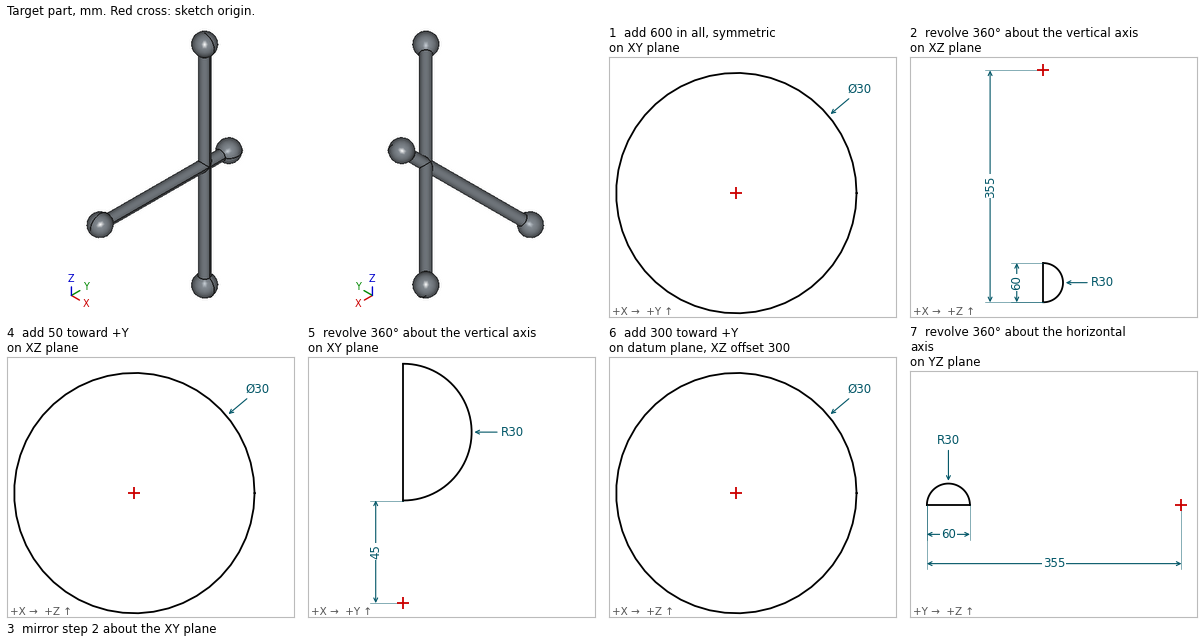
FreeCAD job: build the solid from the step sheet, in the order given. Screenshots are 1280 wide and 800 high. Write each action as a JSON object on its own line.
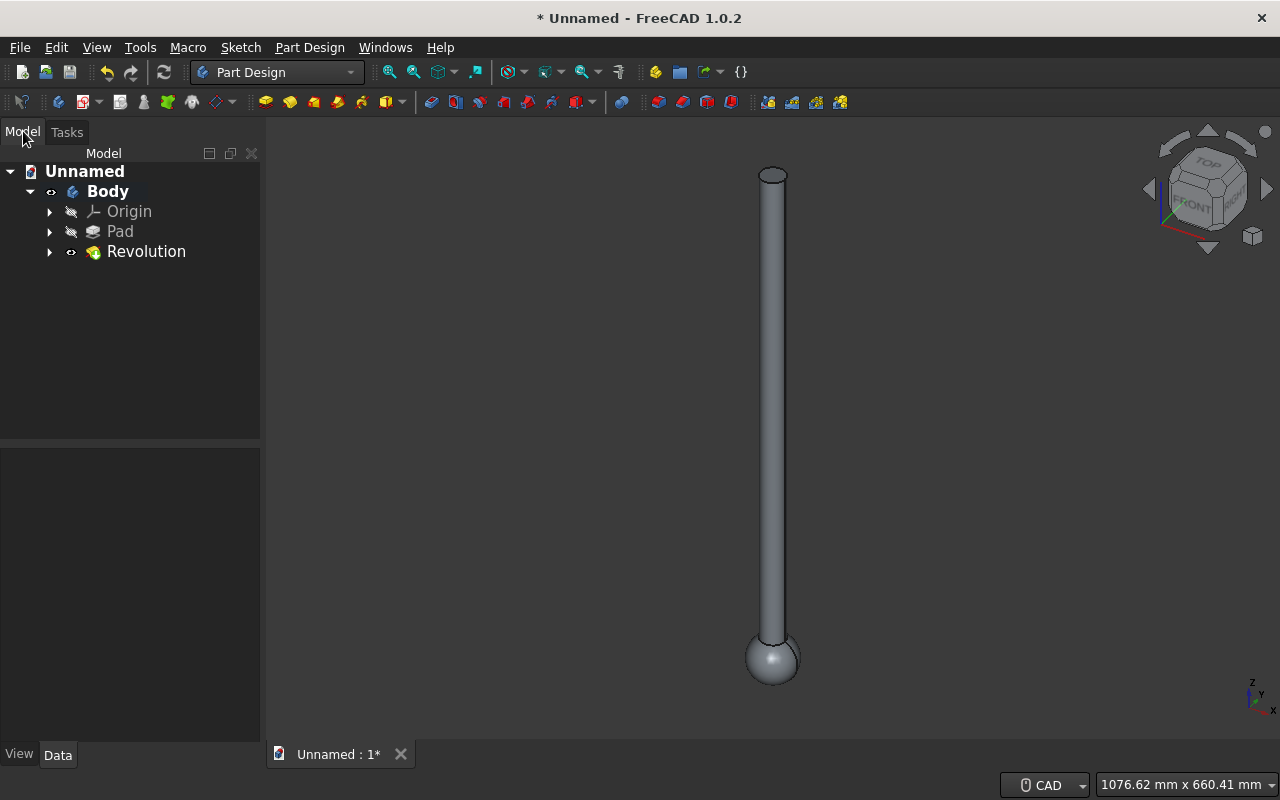
{"action": "left_click", "coordinate": [116, 252]}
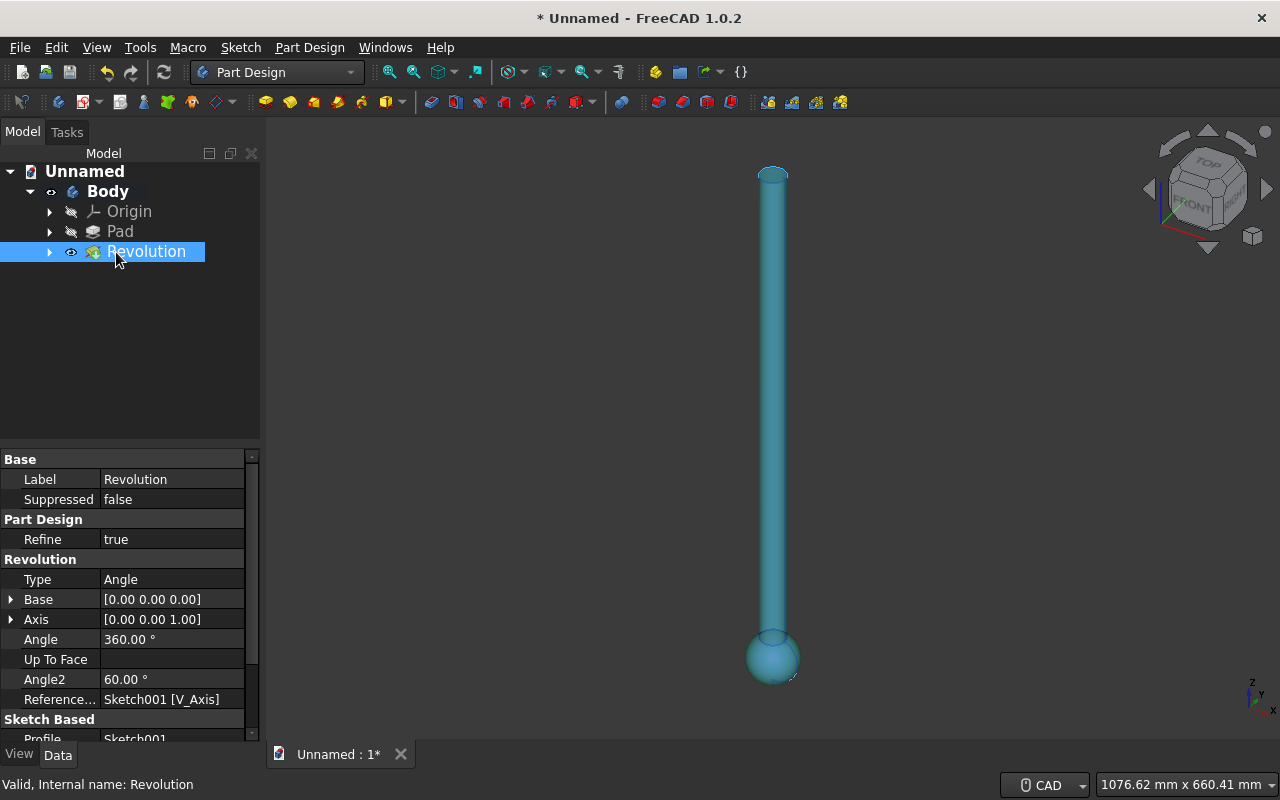
{"action": "left_click", "coordinate": [768, 102]}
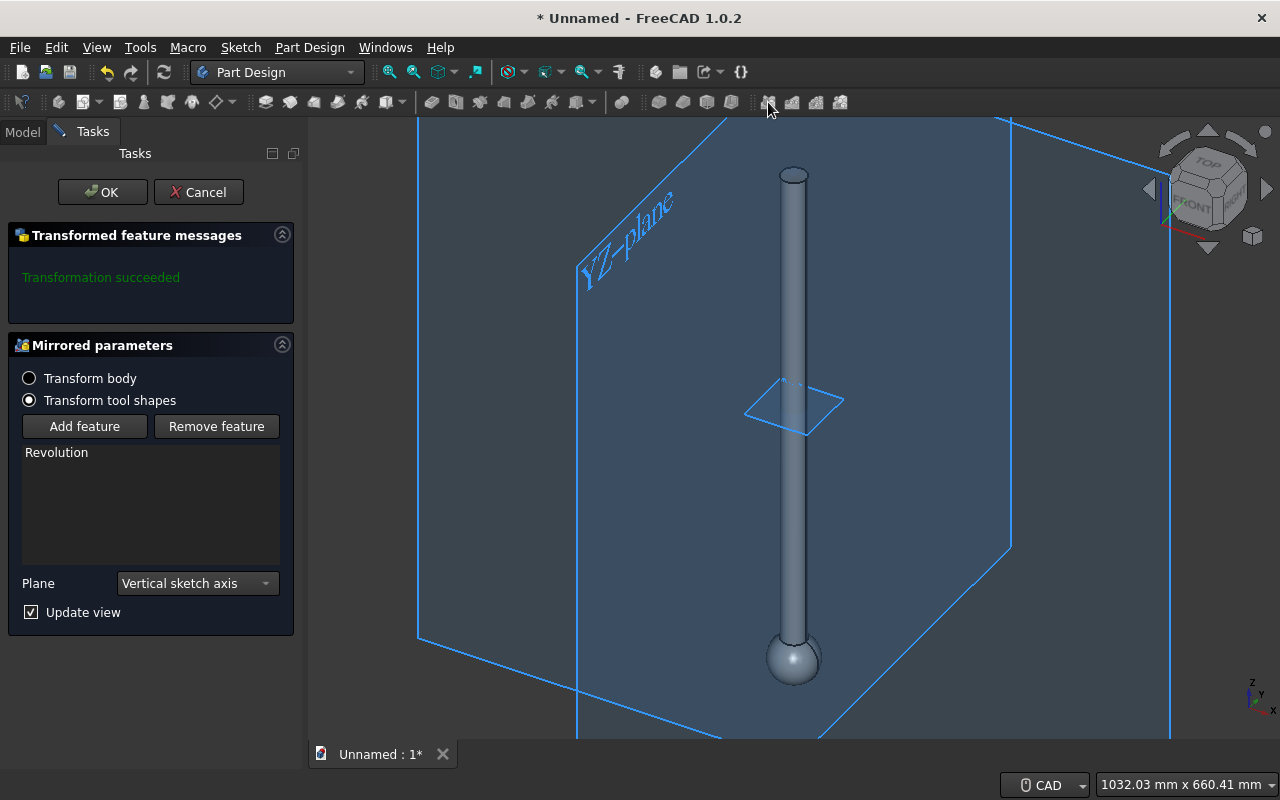
{"action": "left_click", "coordinate": [198, 584]}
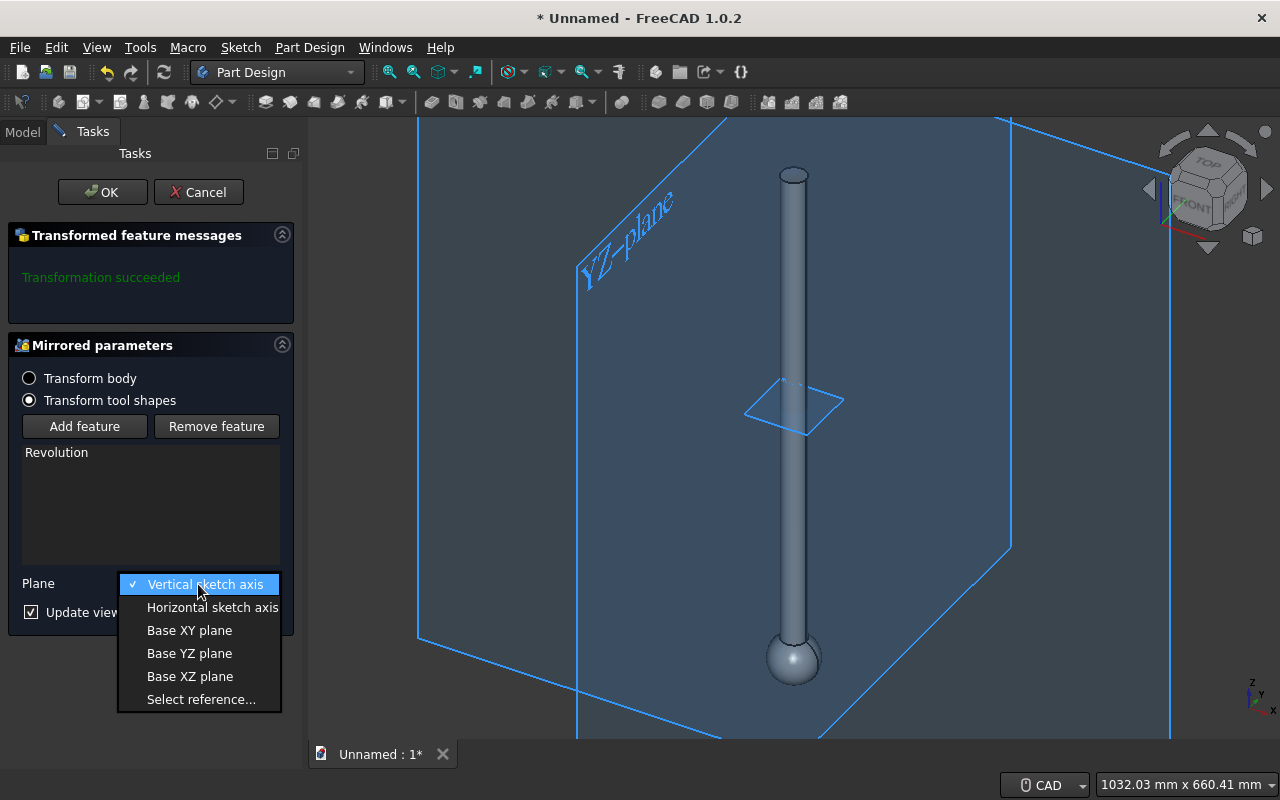
{"action": "left_click", "coordinate": [198, 630]}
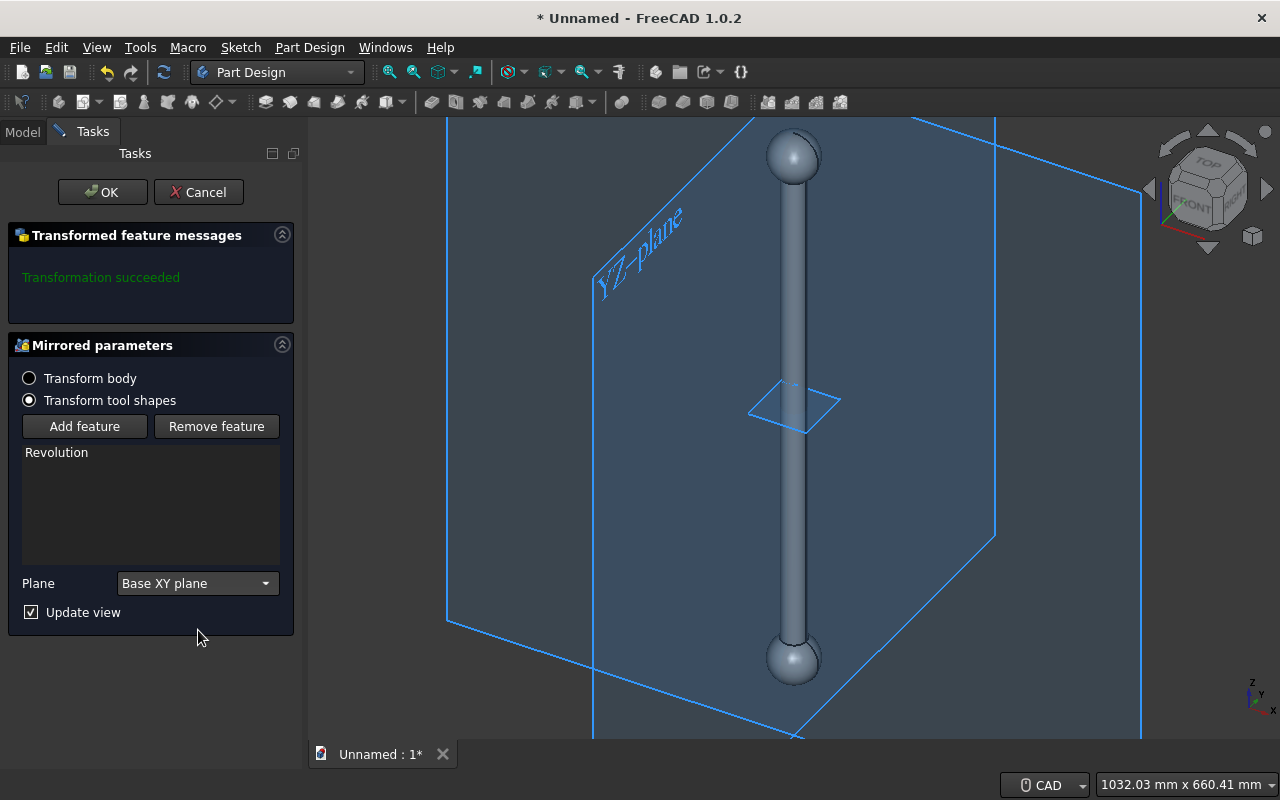
{"action": "left_click", "coordinate": [103, 192]}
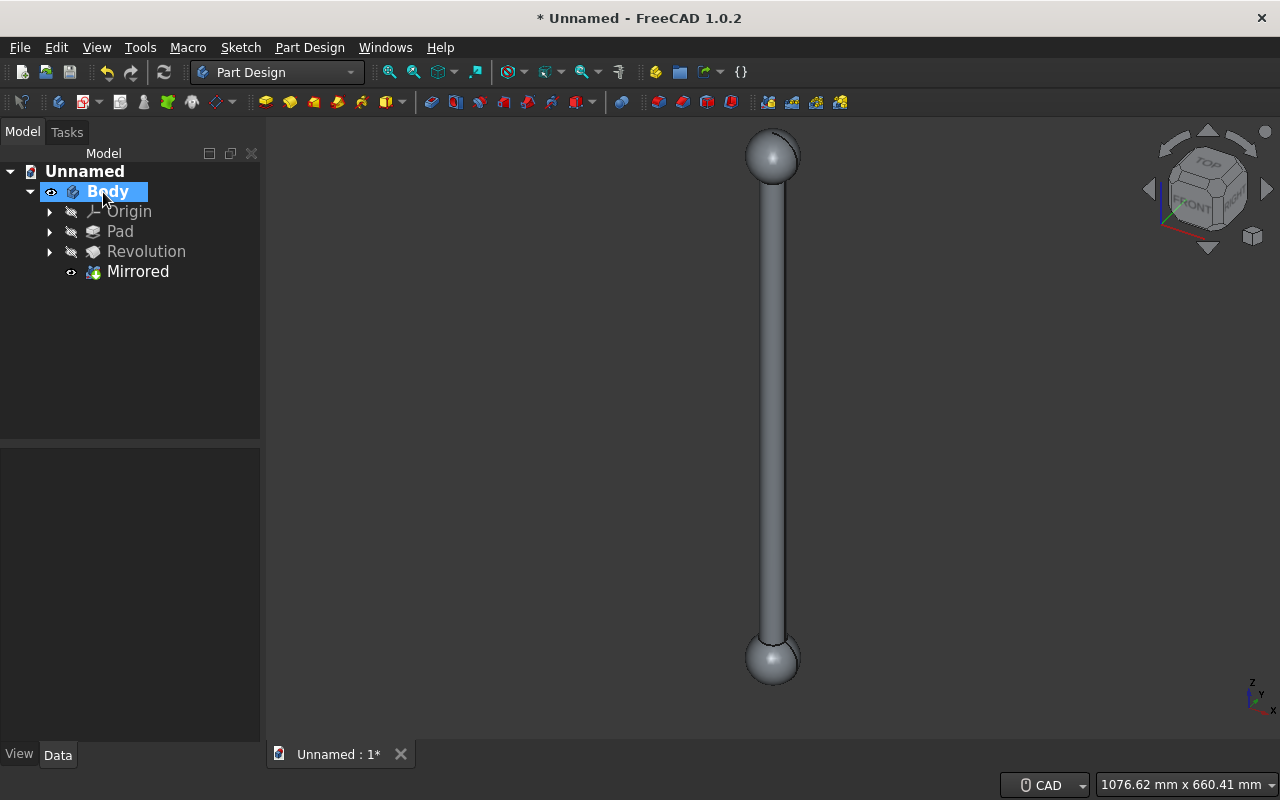
{"action": "left_click", "coordinate": [390, 72]}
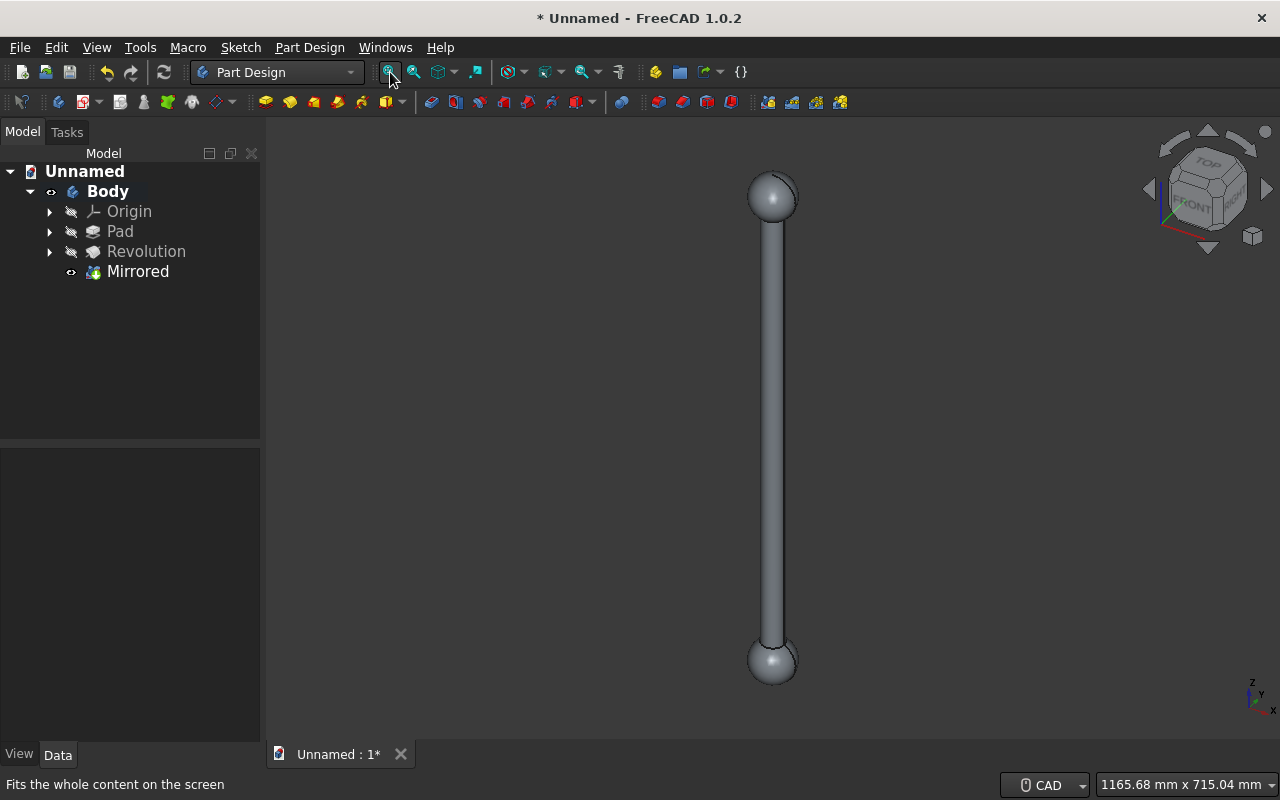
{"action": "left_click", "coordinate": [84, 102]}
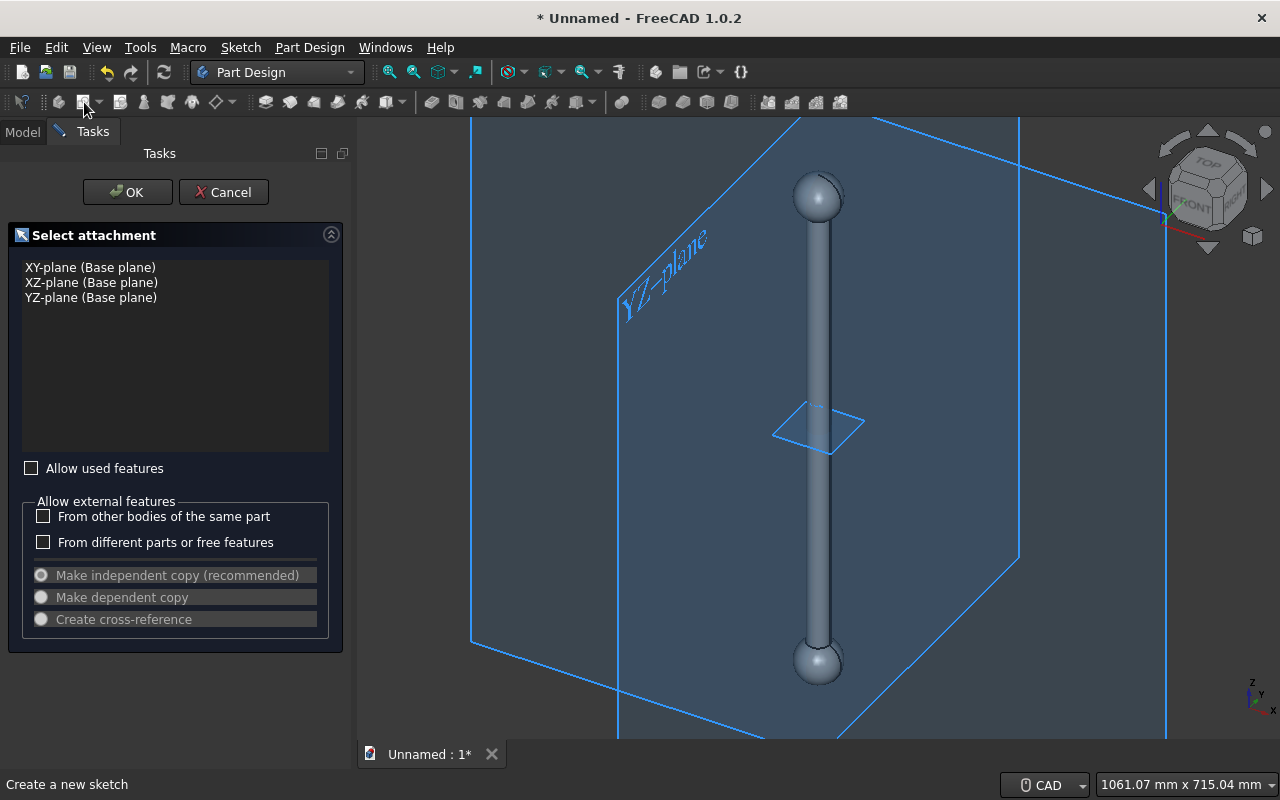
{"action": "left_click", "coordinate": [82, 282]}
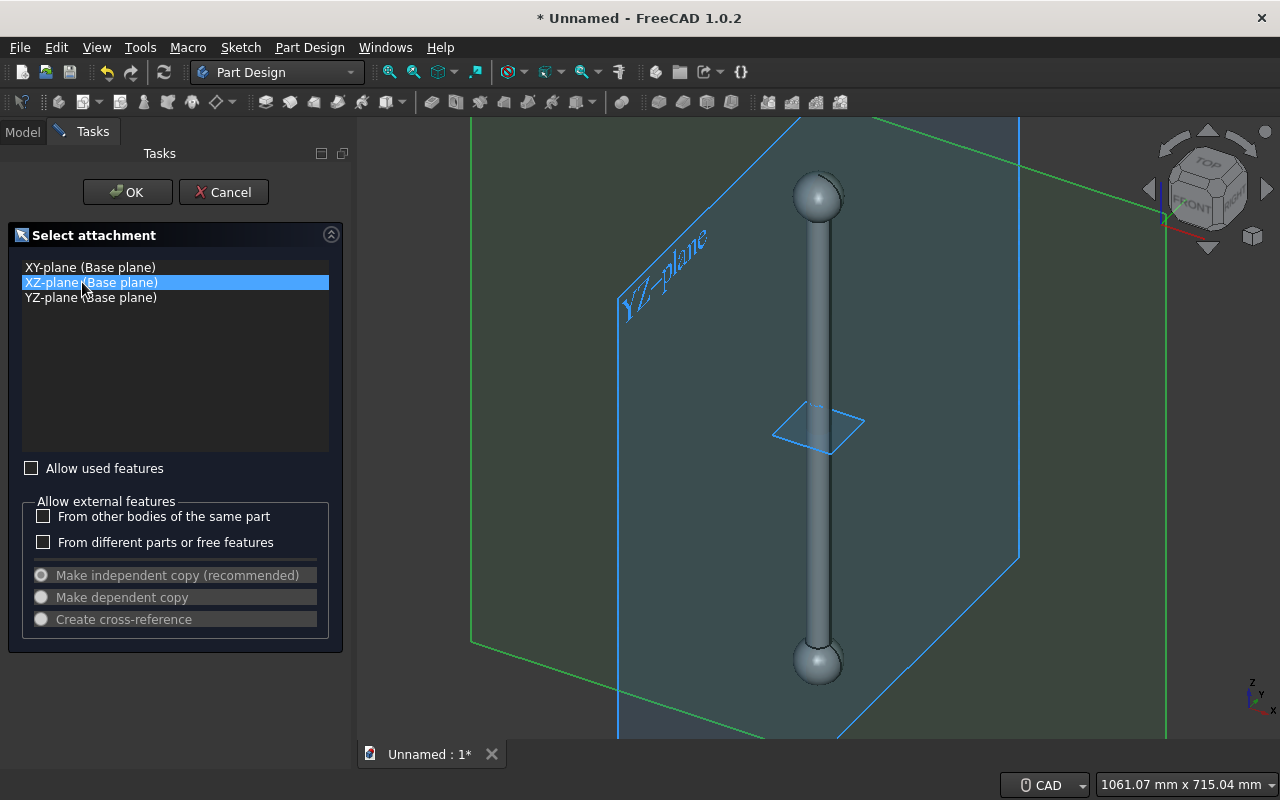
{"action": "left_click", "coordinate": [128, 192]}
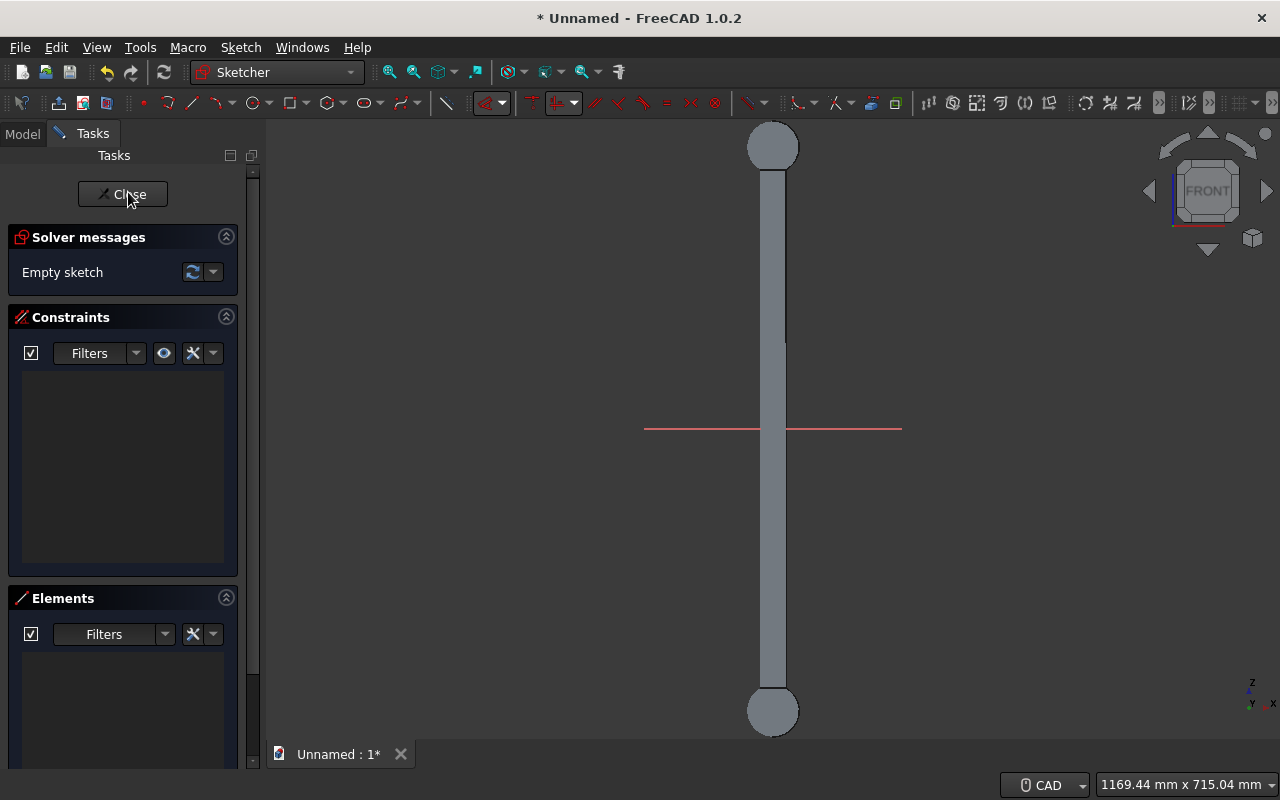
{"action": "left_click", "coordinate": [108, 104]}